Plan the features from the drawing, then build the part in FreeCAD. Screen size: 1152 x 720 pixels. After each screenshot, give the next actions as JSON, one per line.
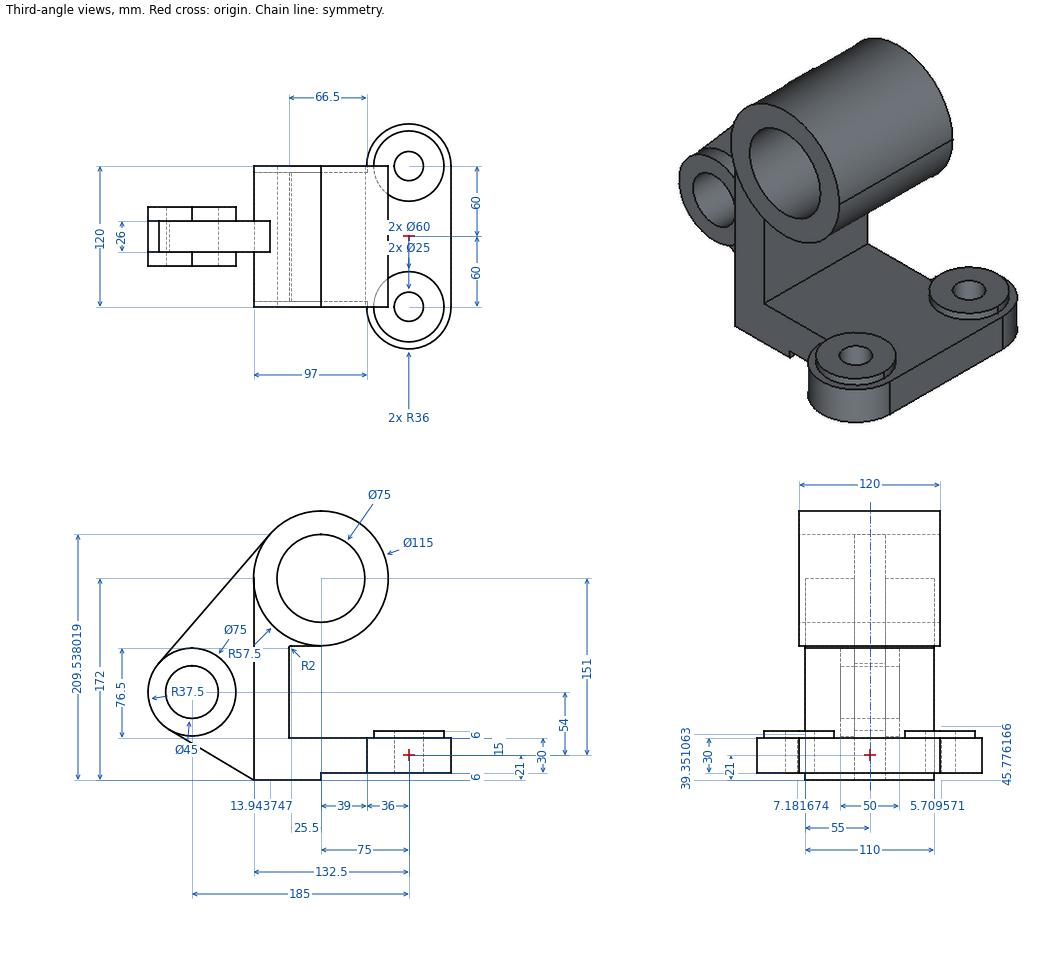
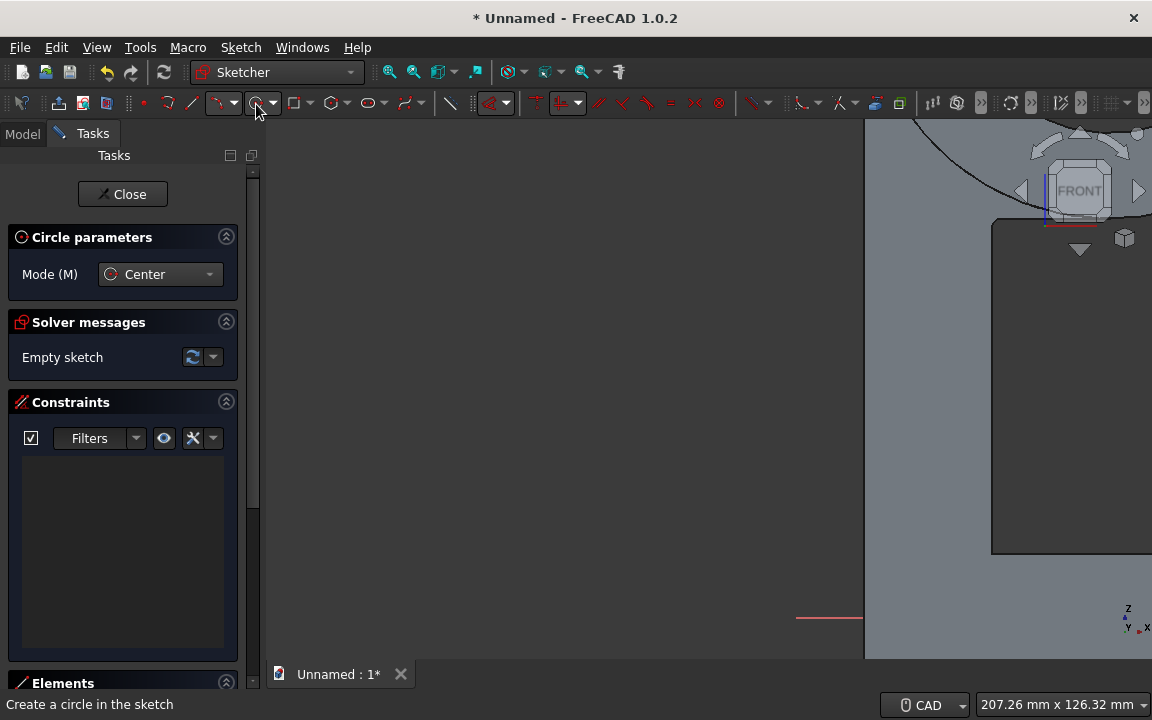
{"action": "left_click", "coordinate": [640, 388]}
{"action": "left_click", "coordinate": [753, 274]}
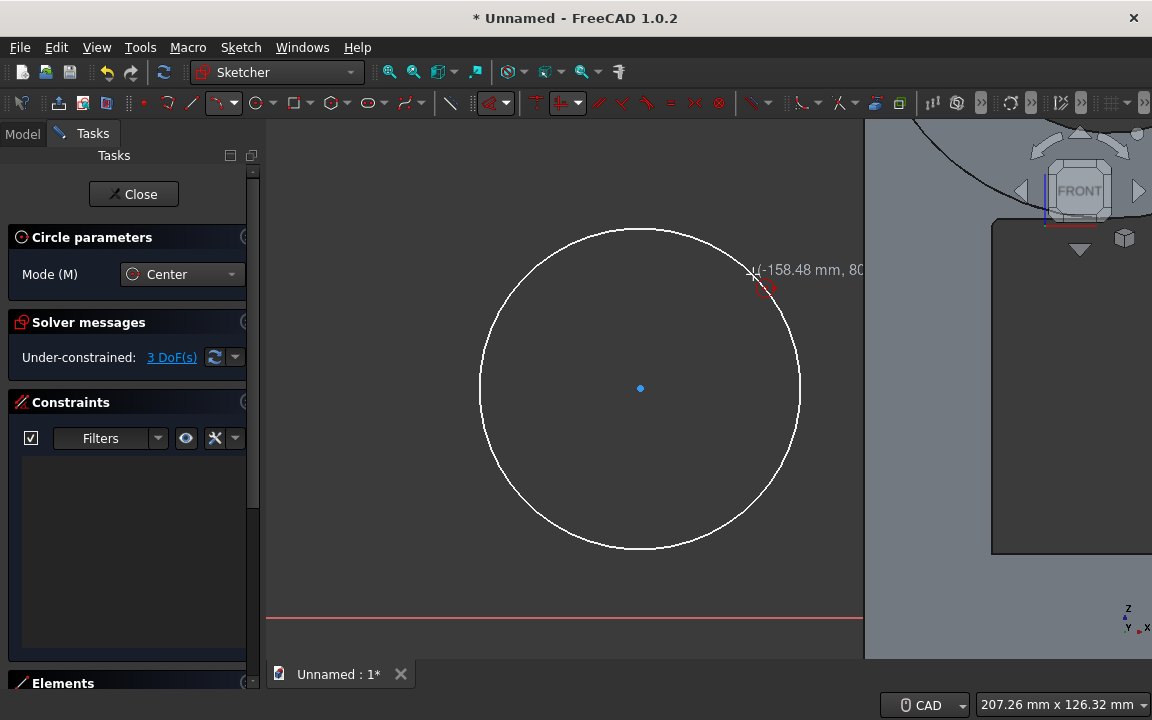
{"action": "left_click", "coordinate": [640, 389]}
{"action": "left_click", "coordinate": [708, 320]}
{"action": "key", "text": "Escape"}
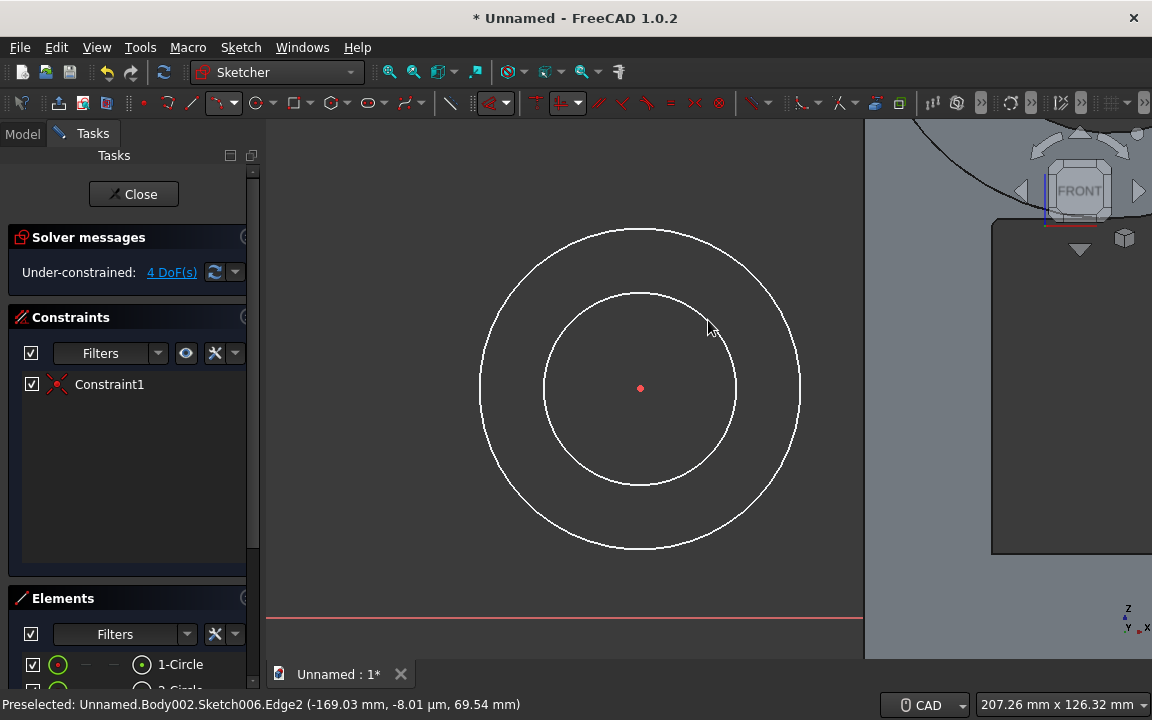
{"action": "left_click", "coordinate": [753, 275]}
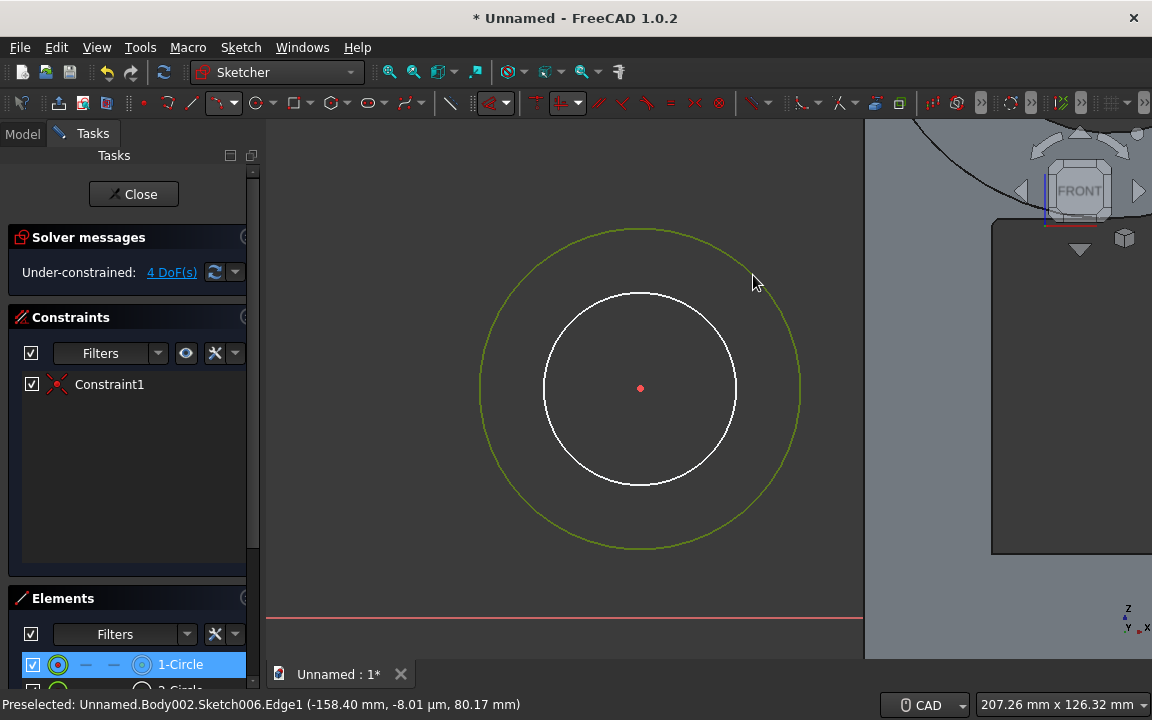
{"action": "key", "text": "k o"}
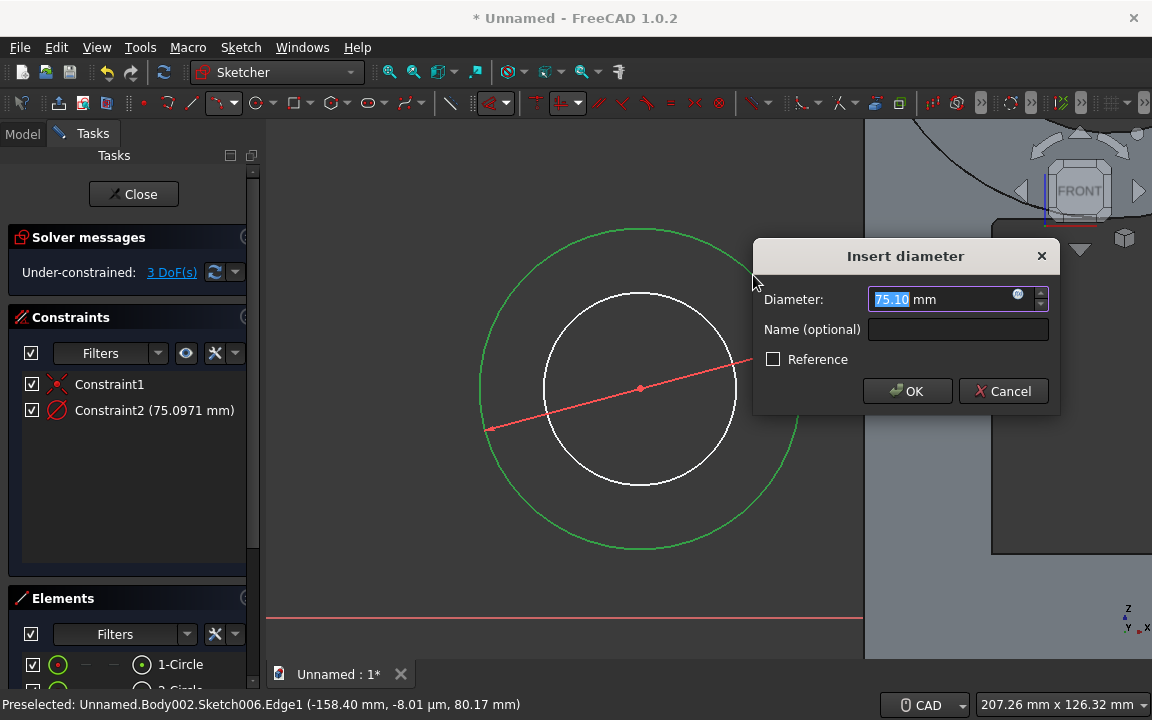
{"action": "type", "text": "75"}
{"action": "key", "text": "Return"}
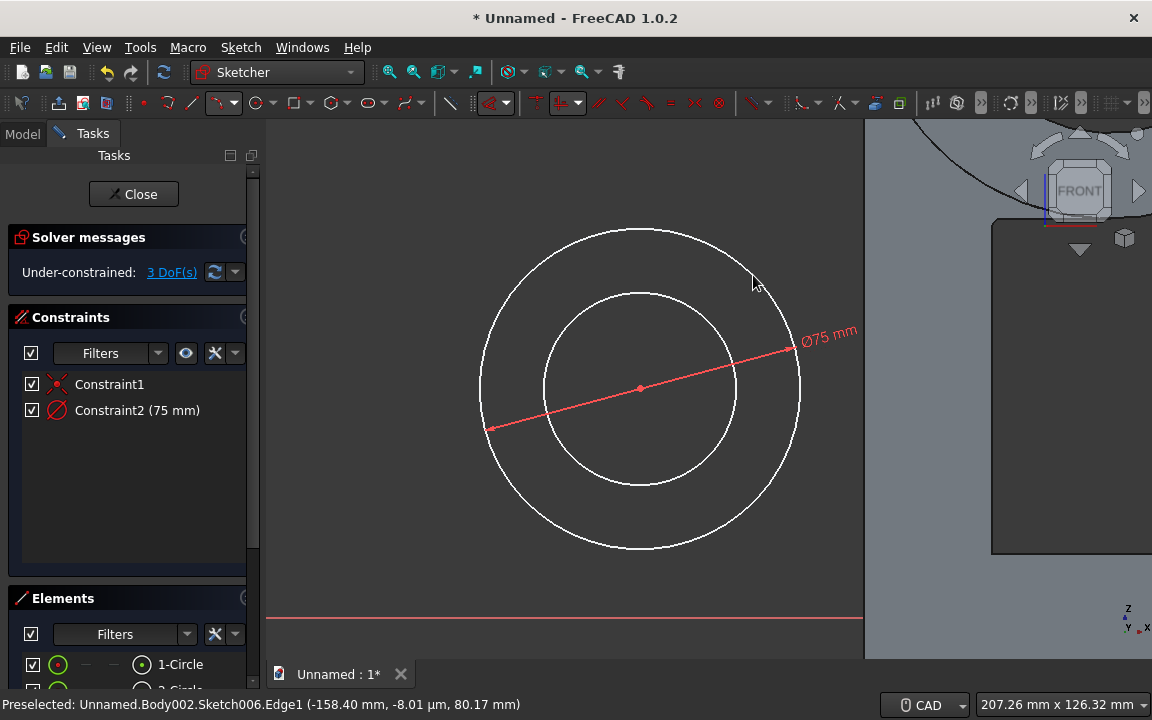
{"action": "left_click", "coordinate": [708, 321]}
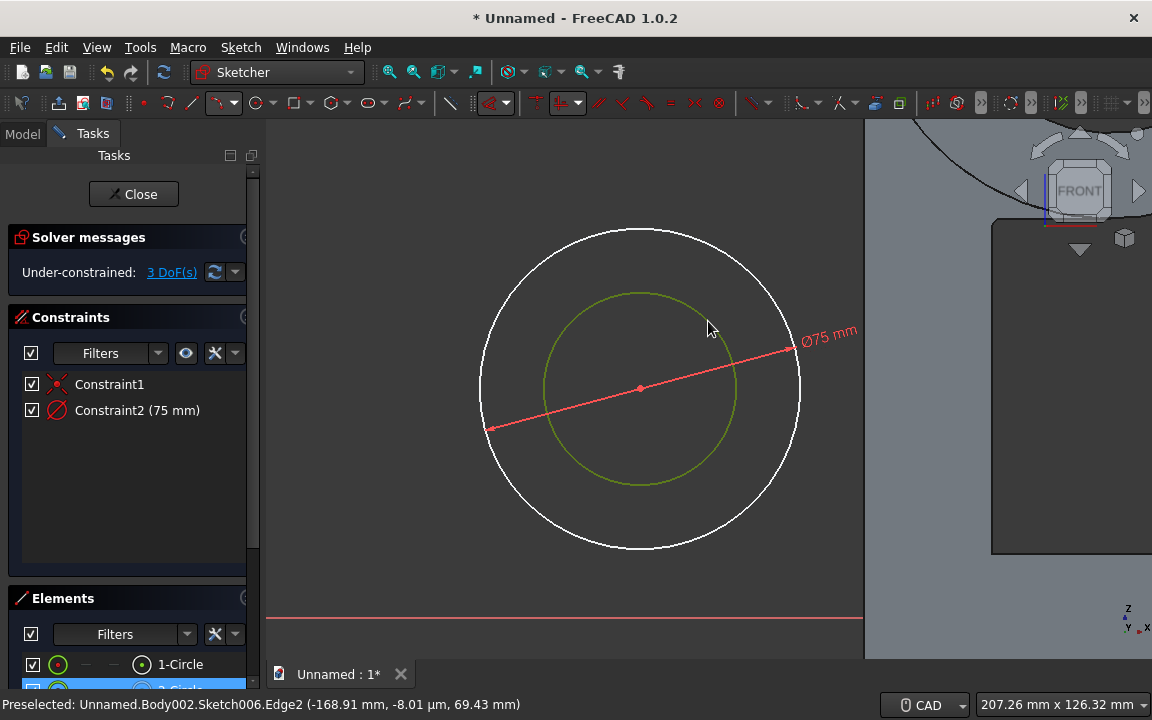
{"action": "key", "text": "k o"}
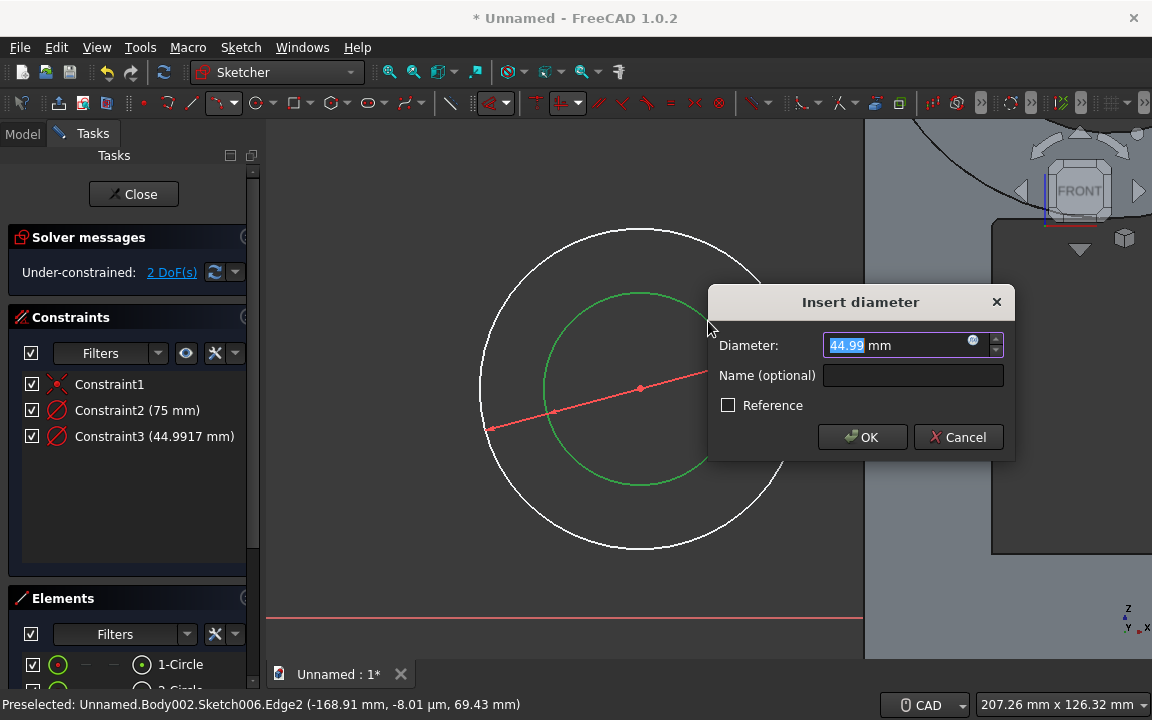
{"action": "type", "text": "45"}
{"action": "key", "text": "Return"}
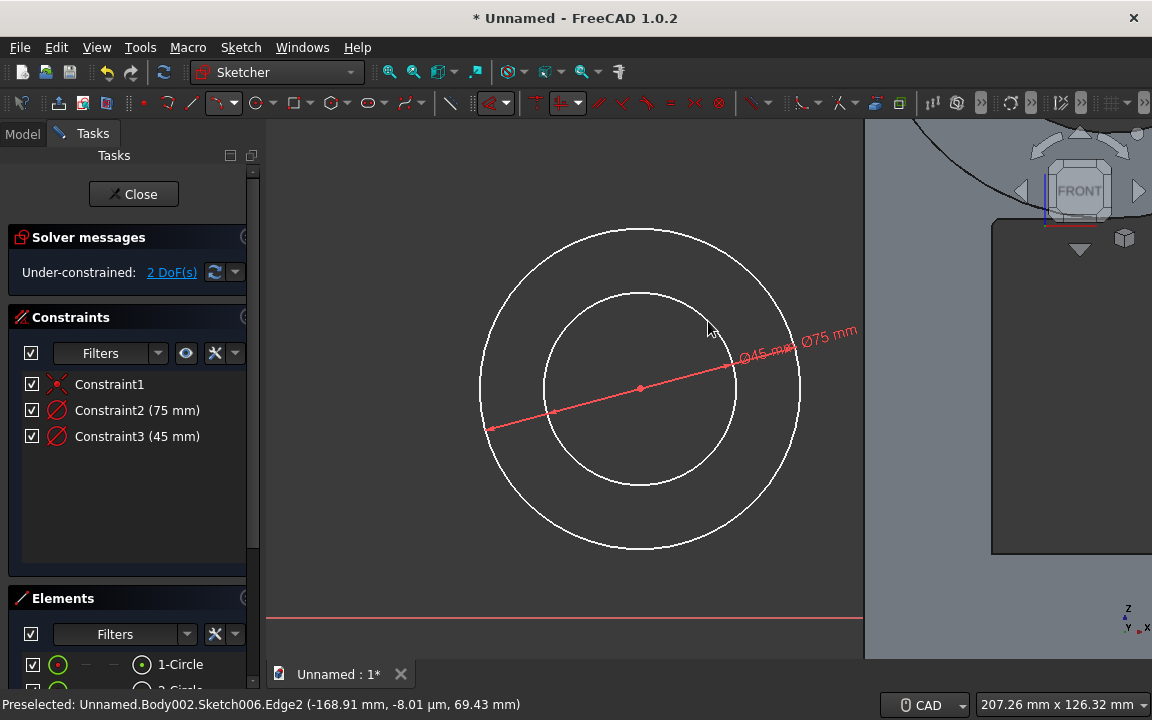
{"action": "left_click", "coordinate": [640, 389]}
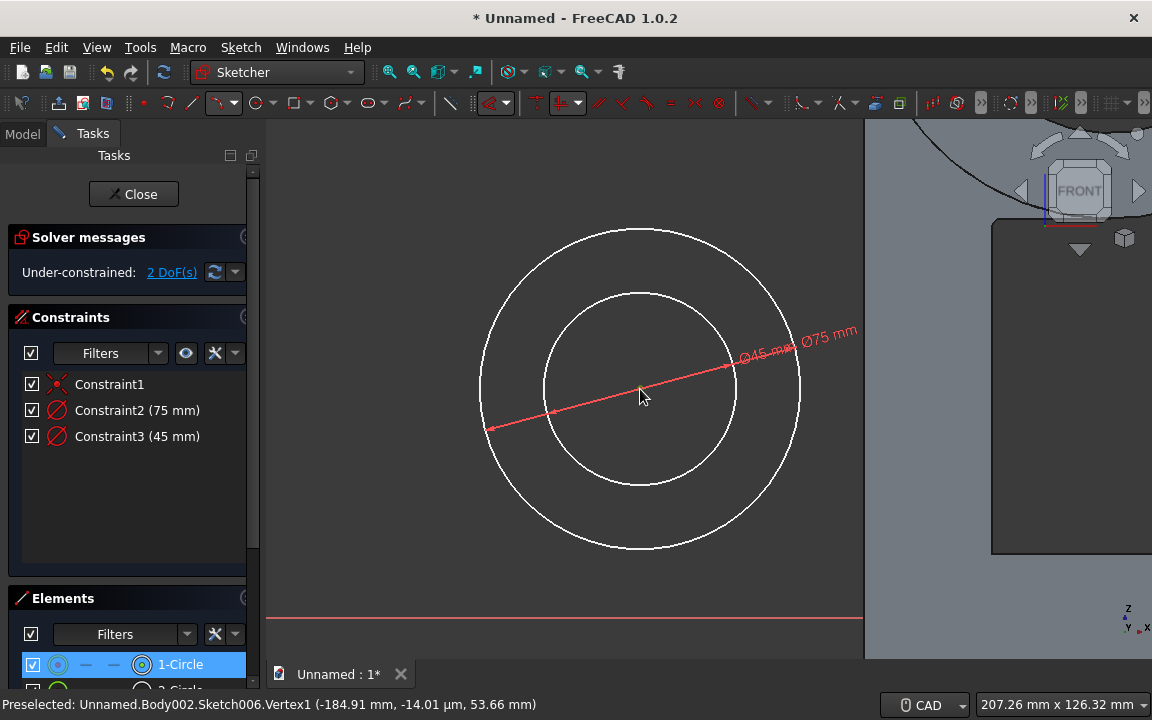
{"action": "key", "text": "i"}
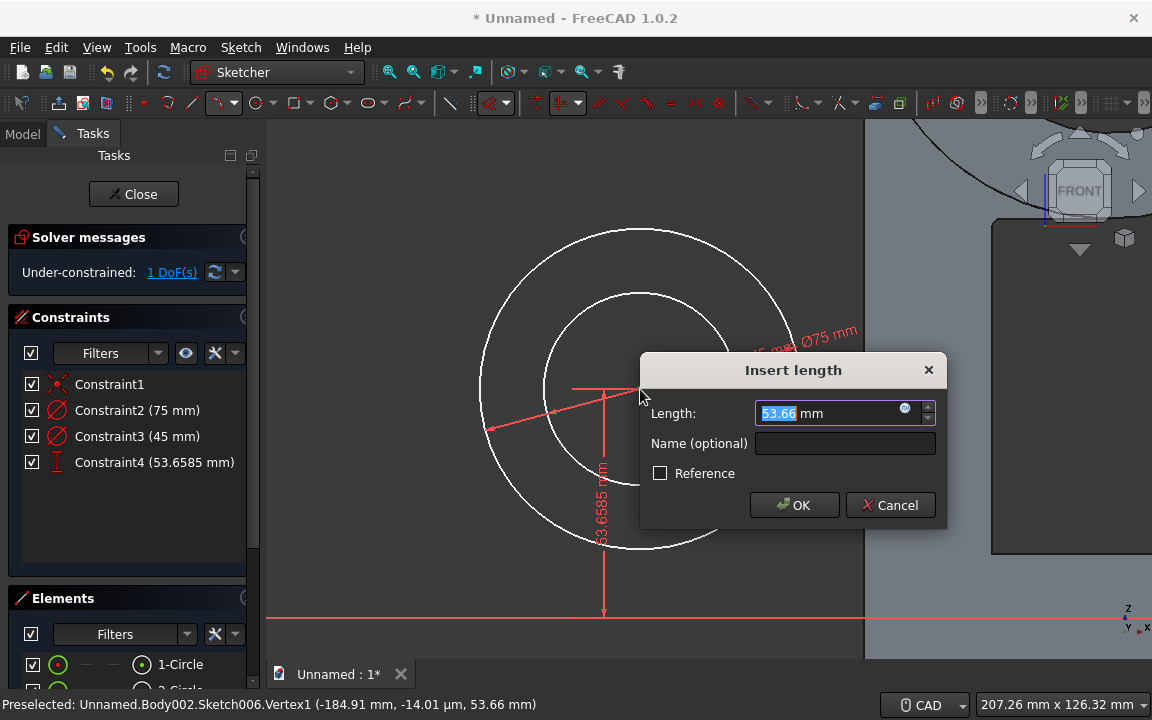
{"action": "type", "text": "54"}
{"action": "key", "text": "Return"}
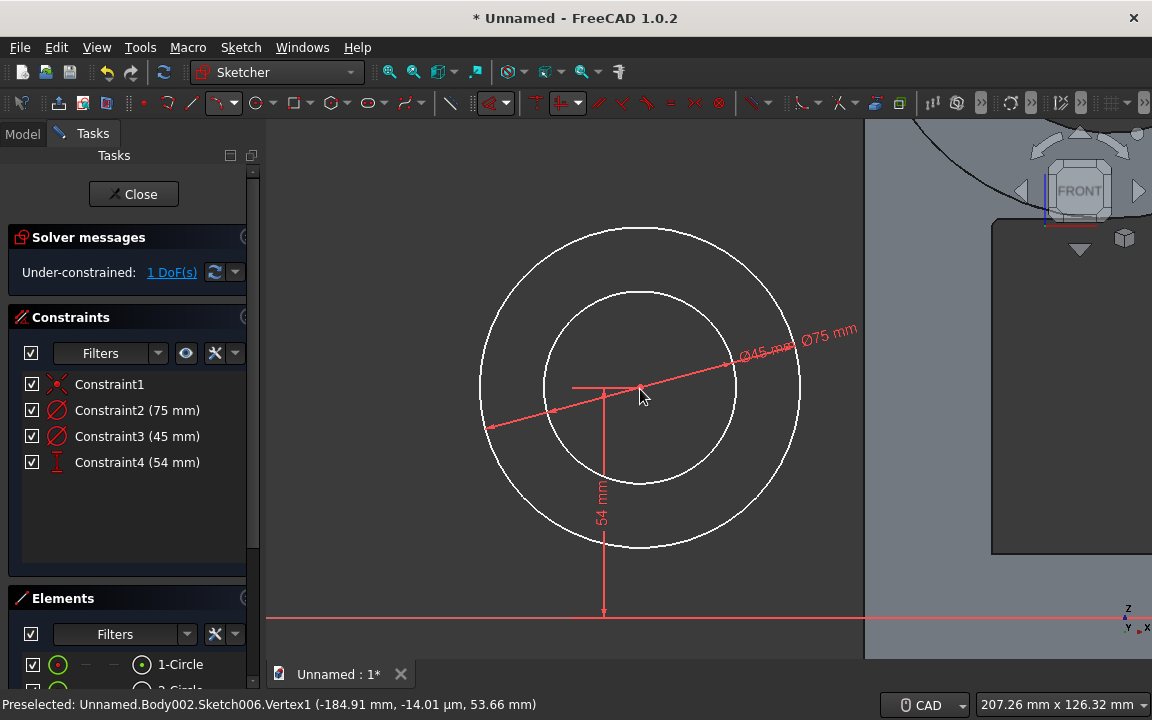
{"action": "left_click", "coordinate": [640, 388]}